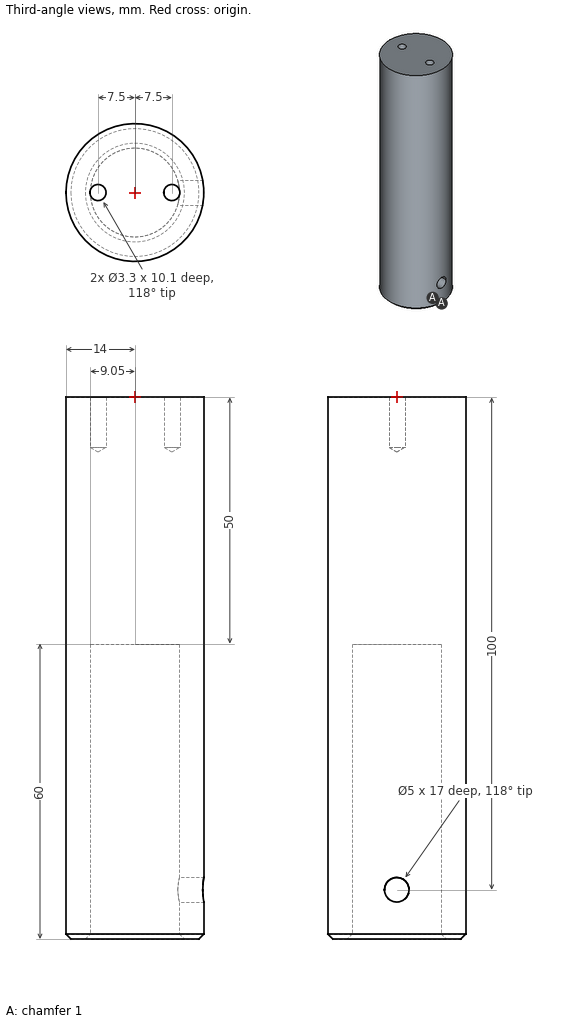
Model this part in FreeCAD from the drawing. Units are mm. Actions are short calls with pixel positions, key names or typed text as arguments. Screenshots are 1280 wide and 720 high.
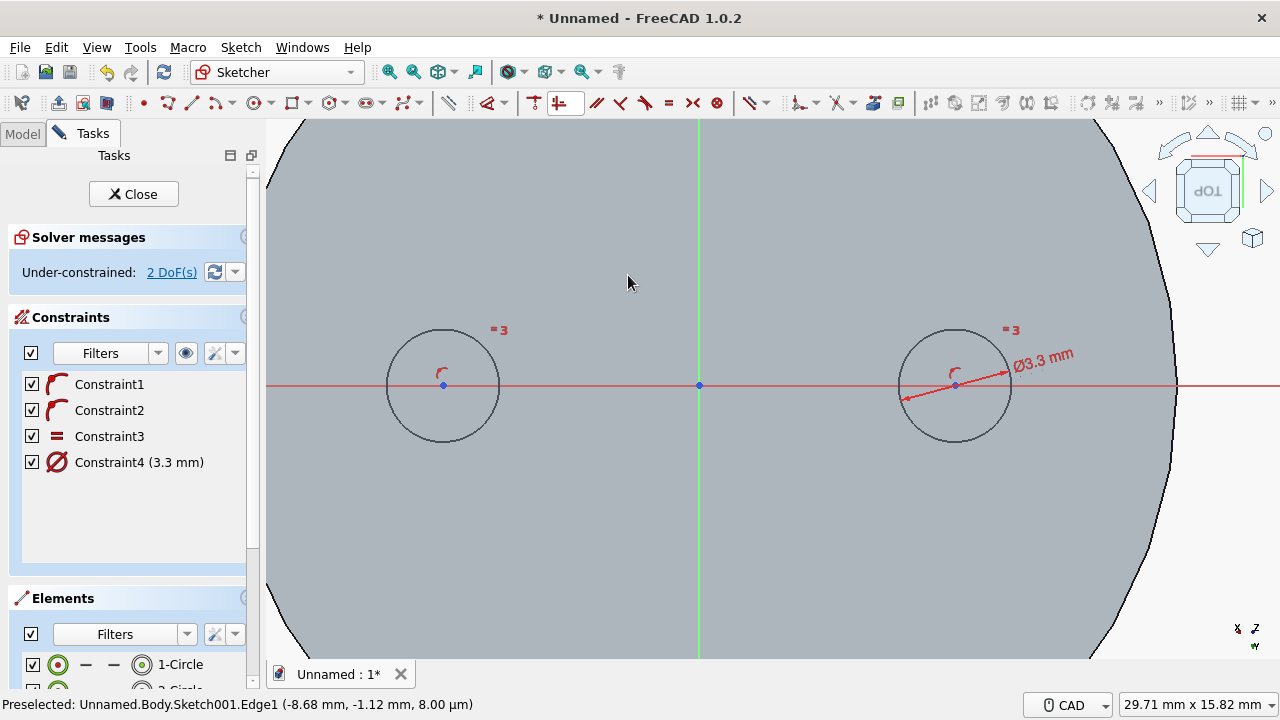
click(955, 386)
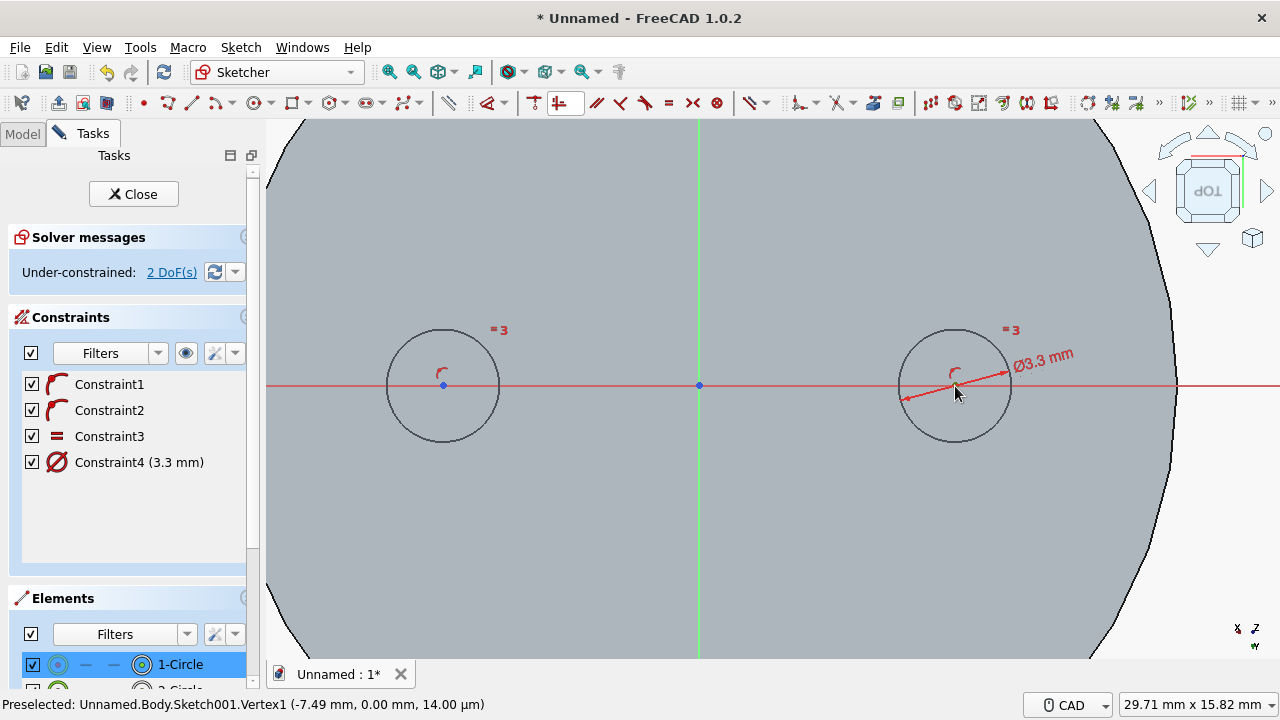
click(506, 104)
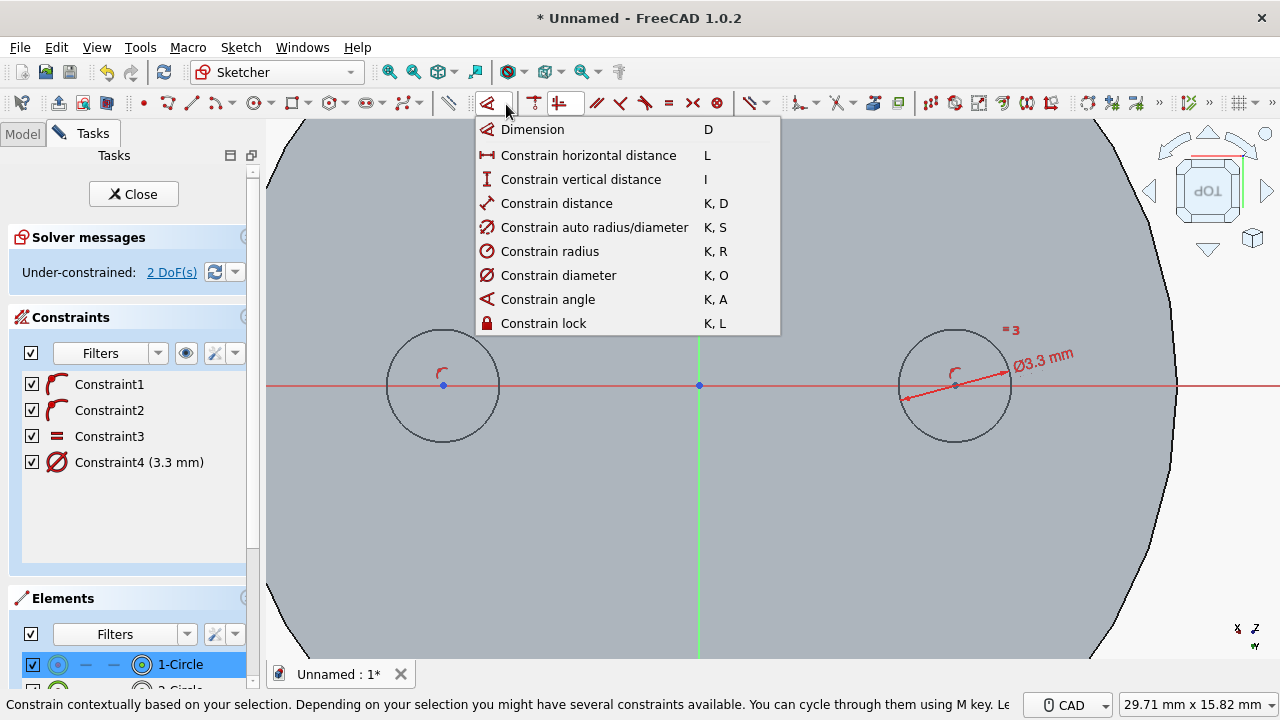
click(628, 155)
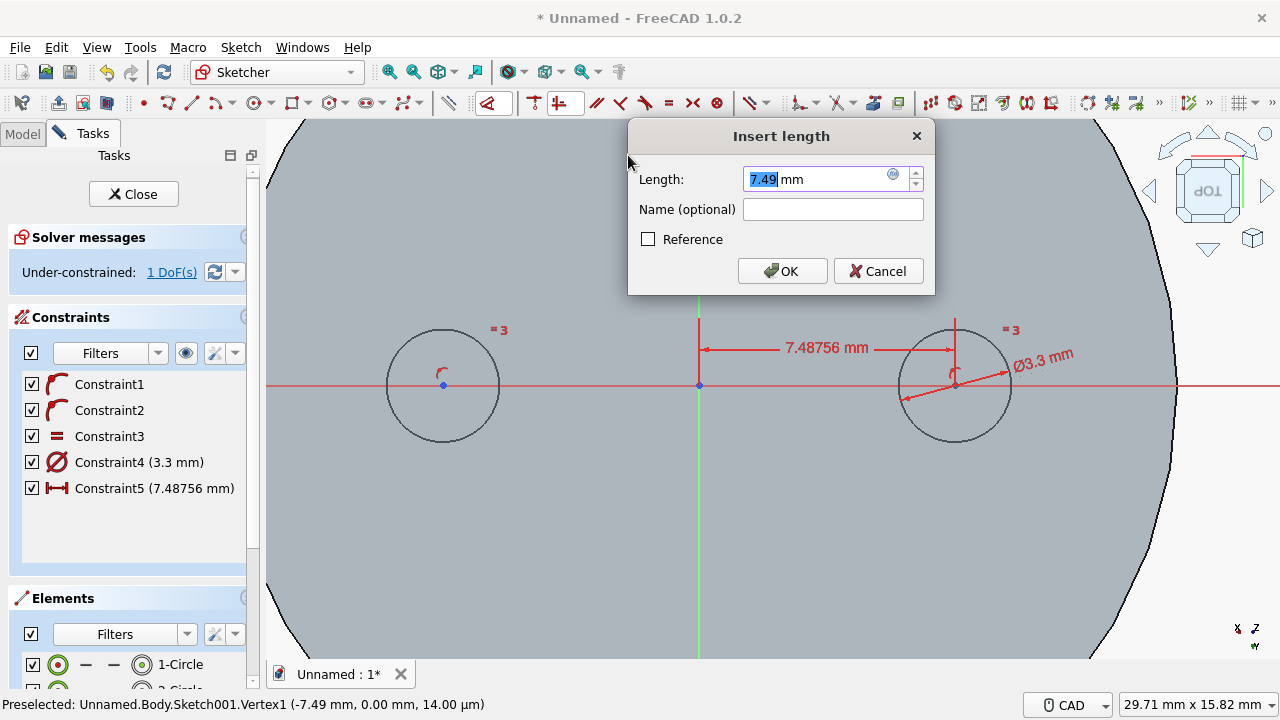
text(7.5)
key(Return)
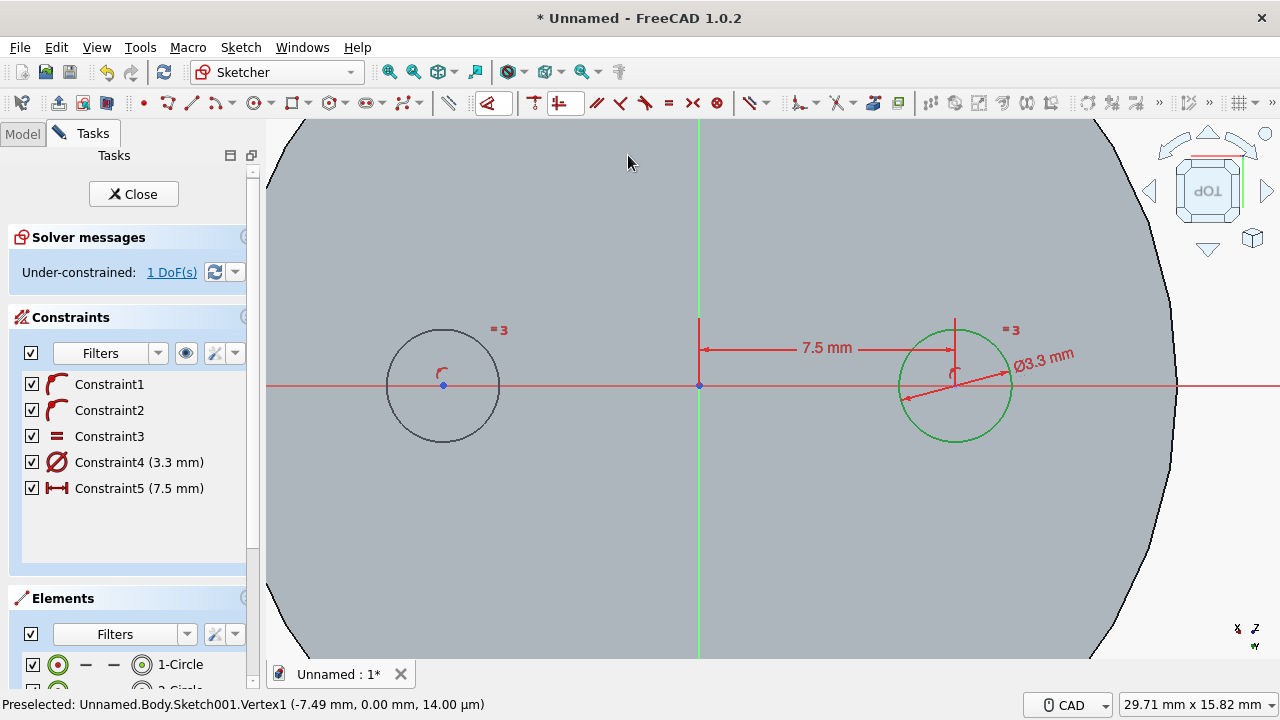
click(443, 386)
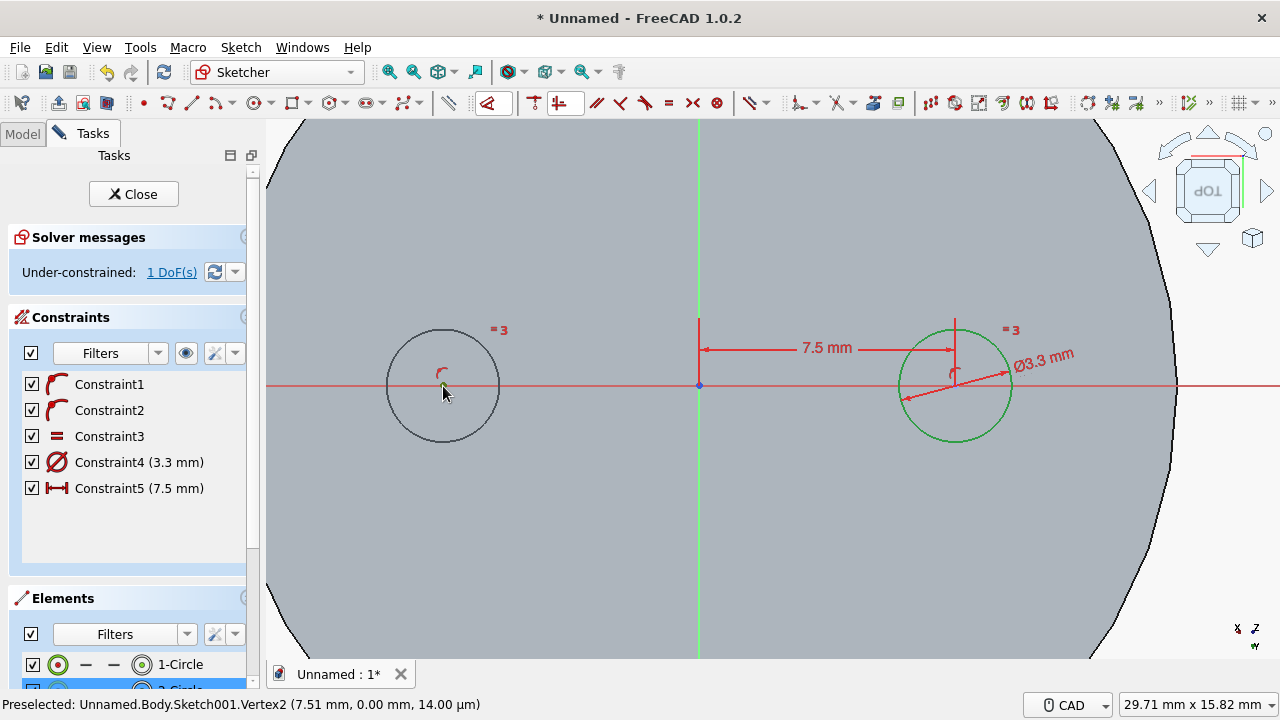
key(l)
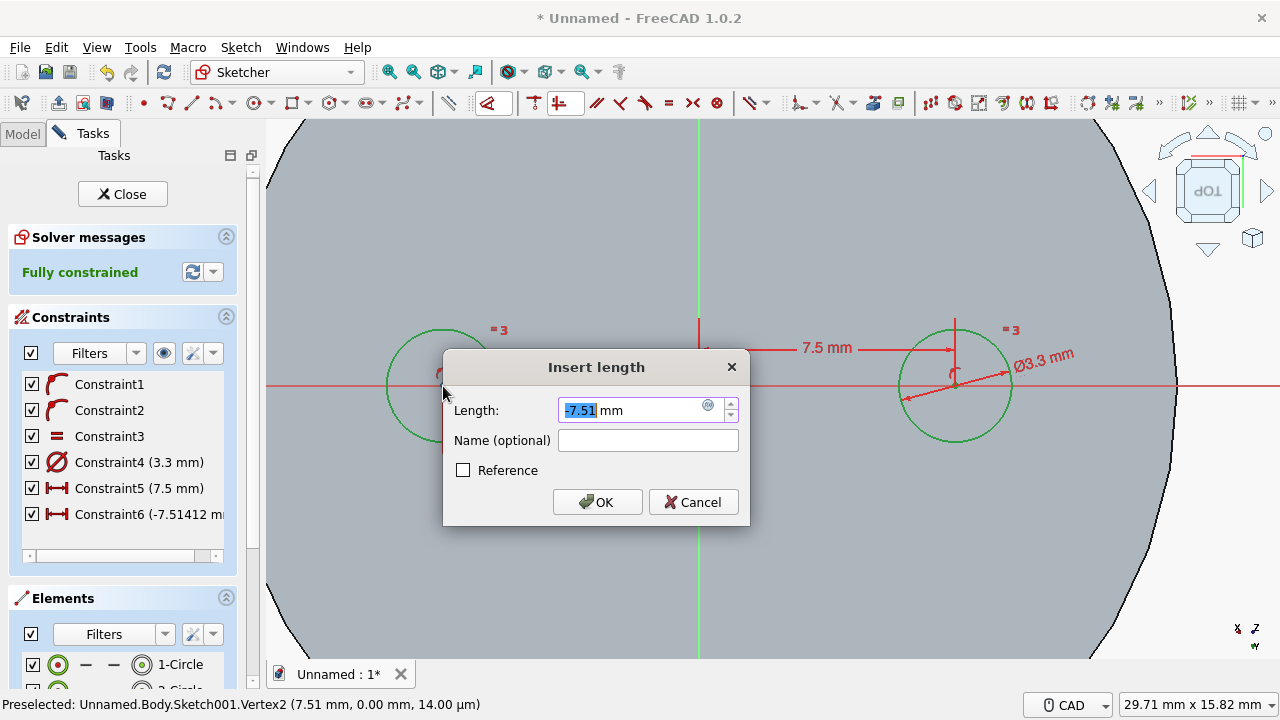
text(-7.5)
key(Return)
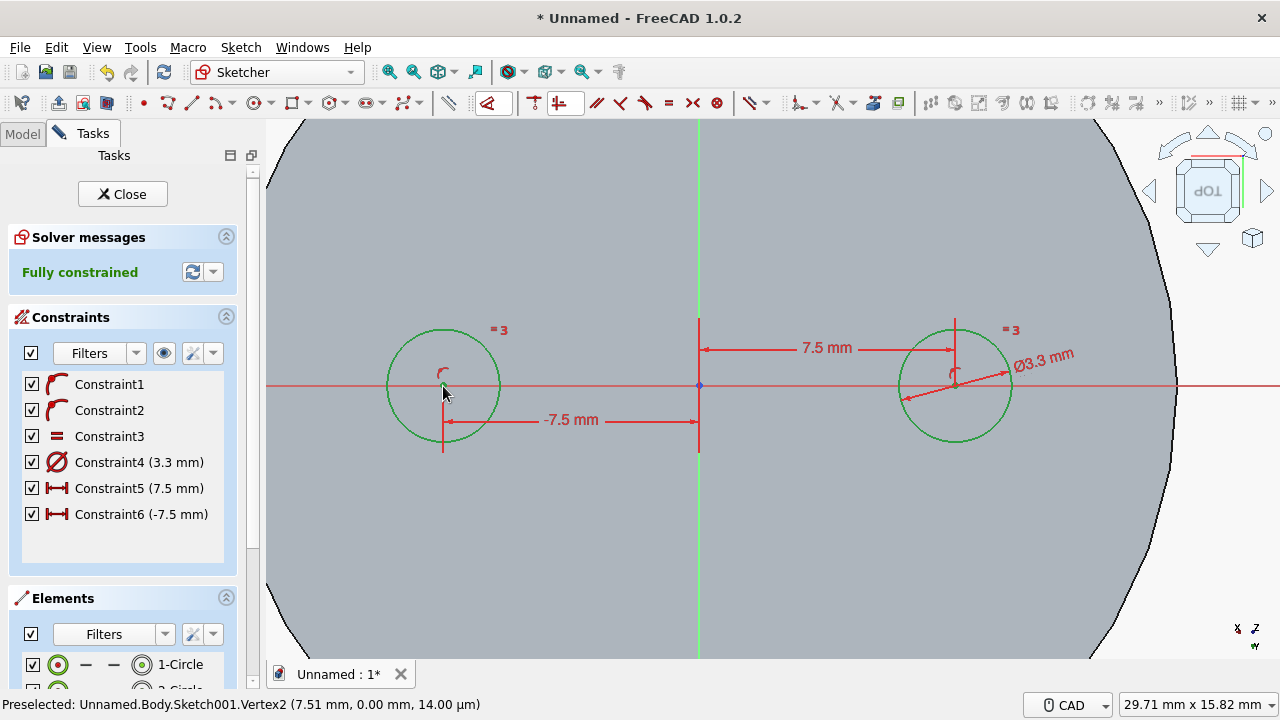
click(123, 194)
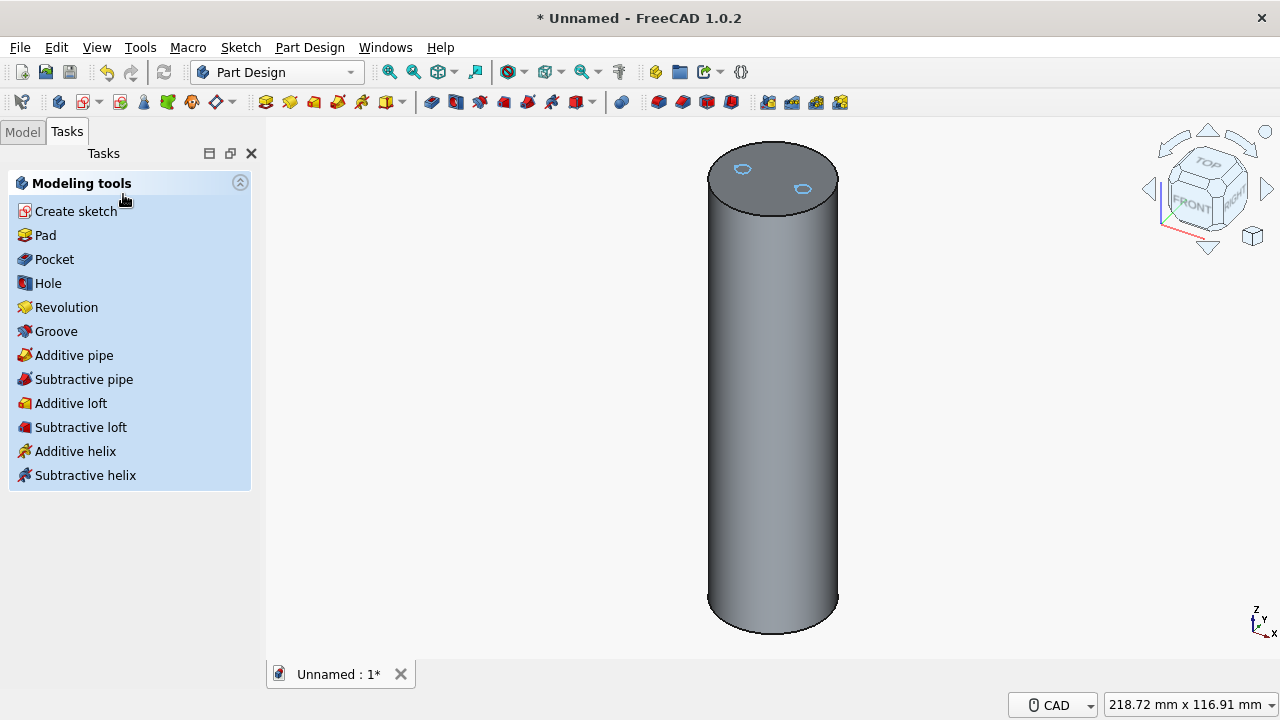
click(456, 102)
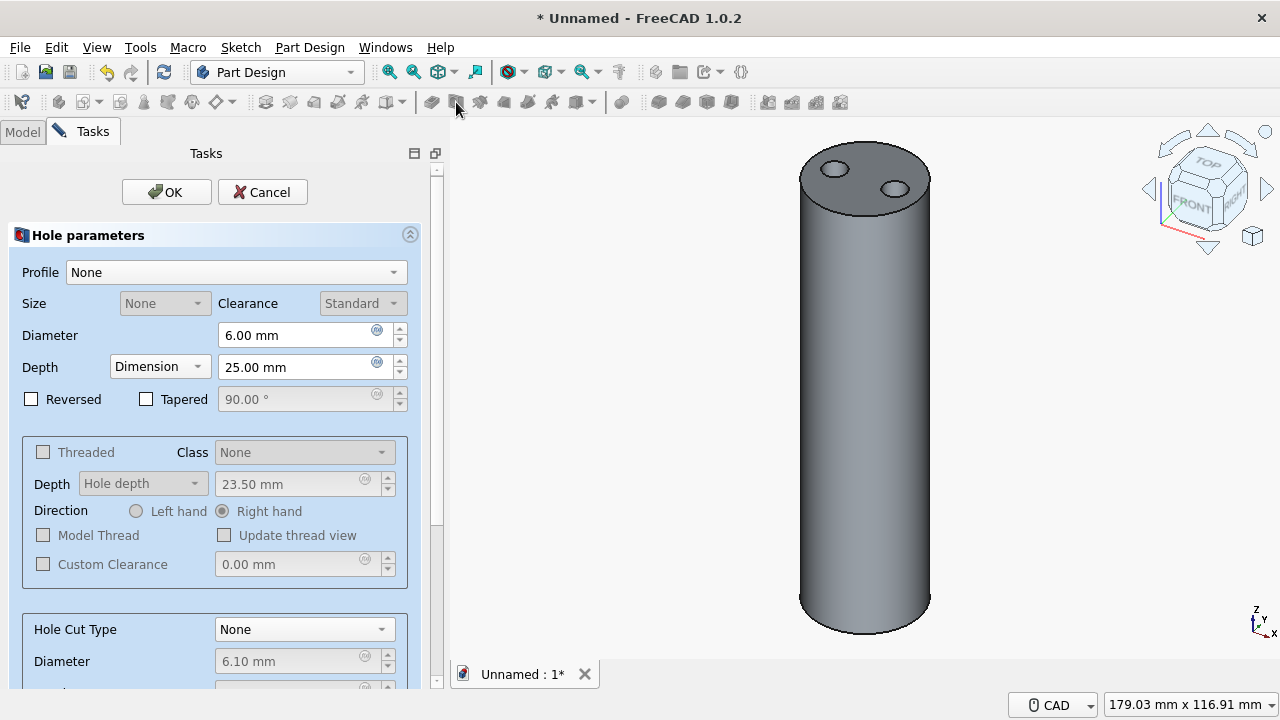
triple_click(305, 335)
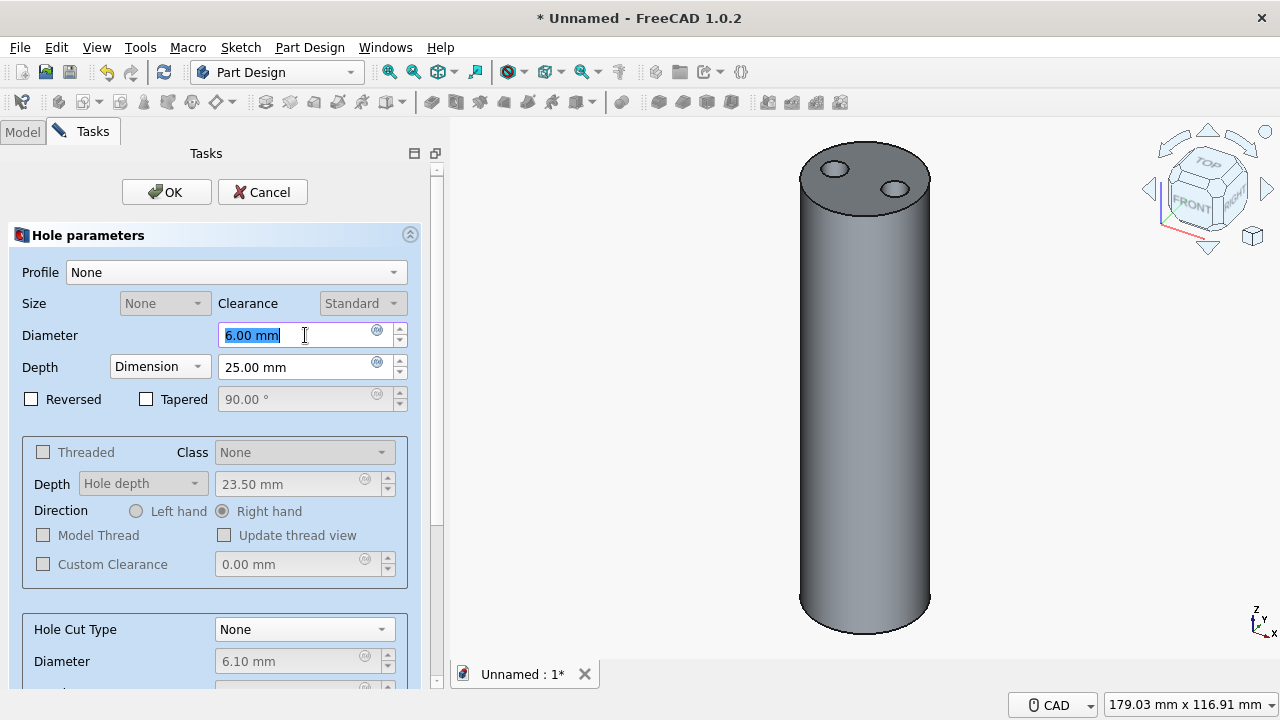
text(3.3)
key(Tab)